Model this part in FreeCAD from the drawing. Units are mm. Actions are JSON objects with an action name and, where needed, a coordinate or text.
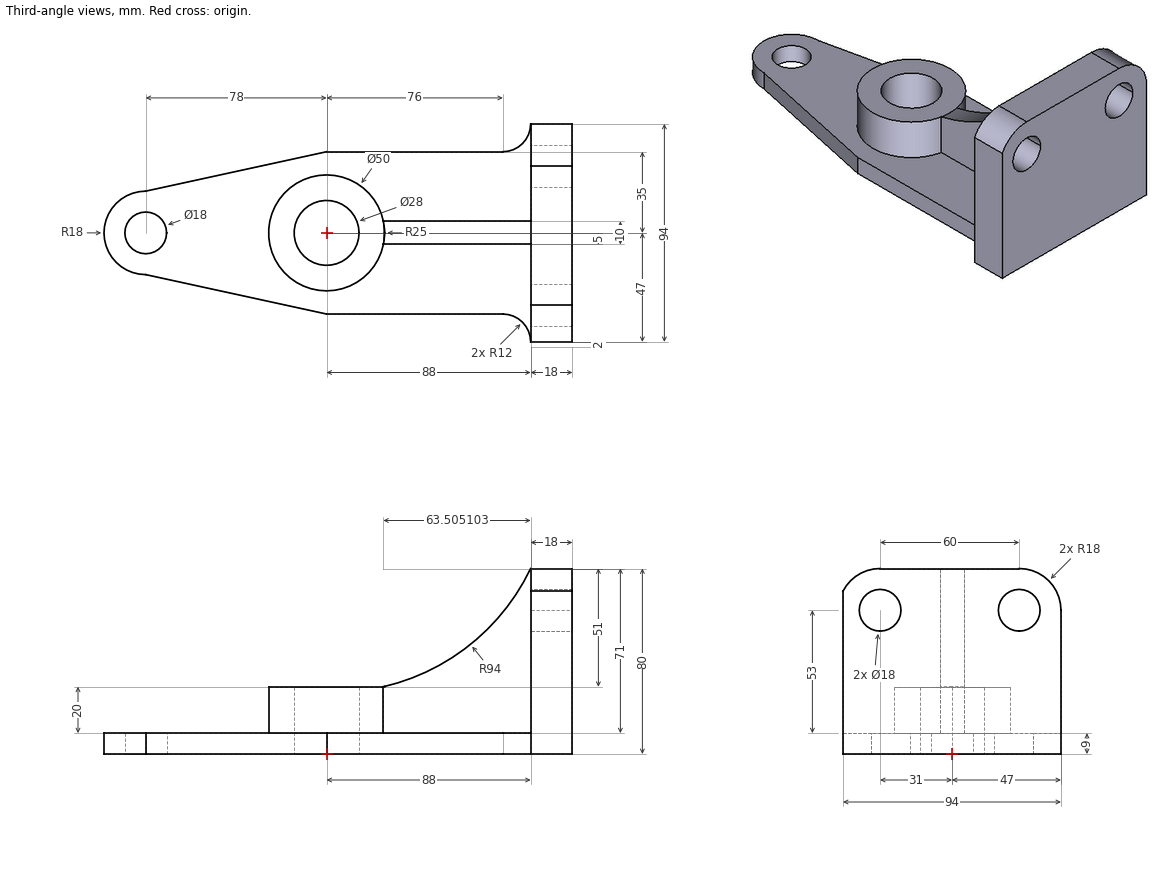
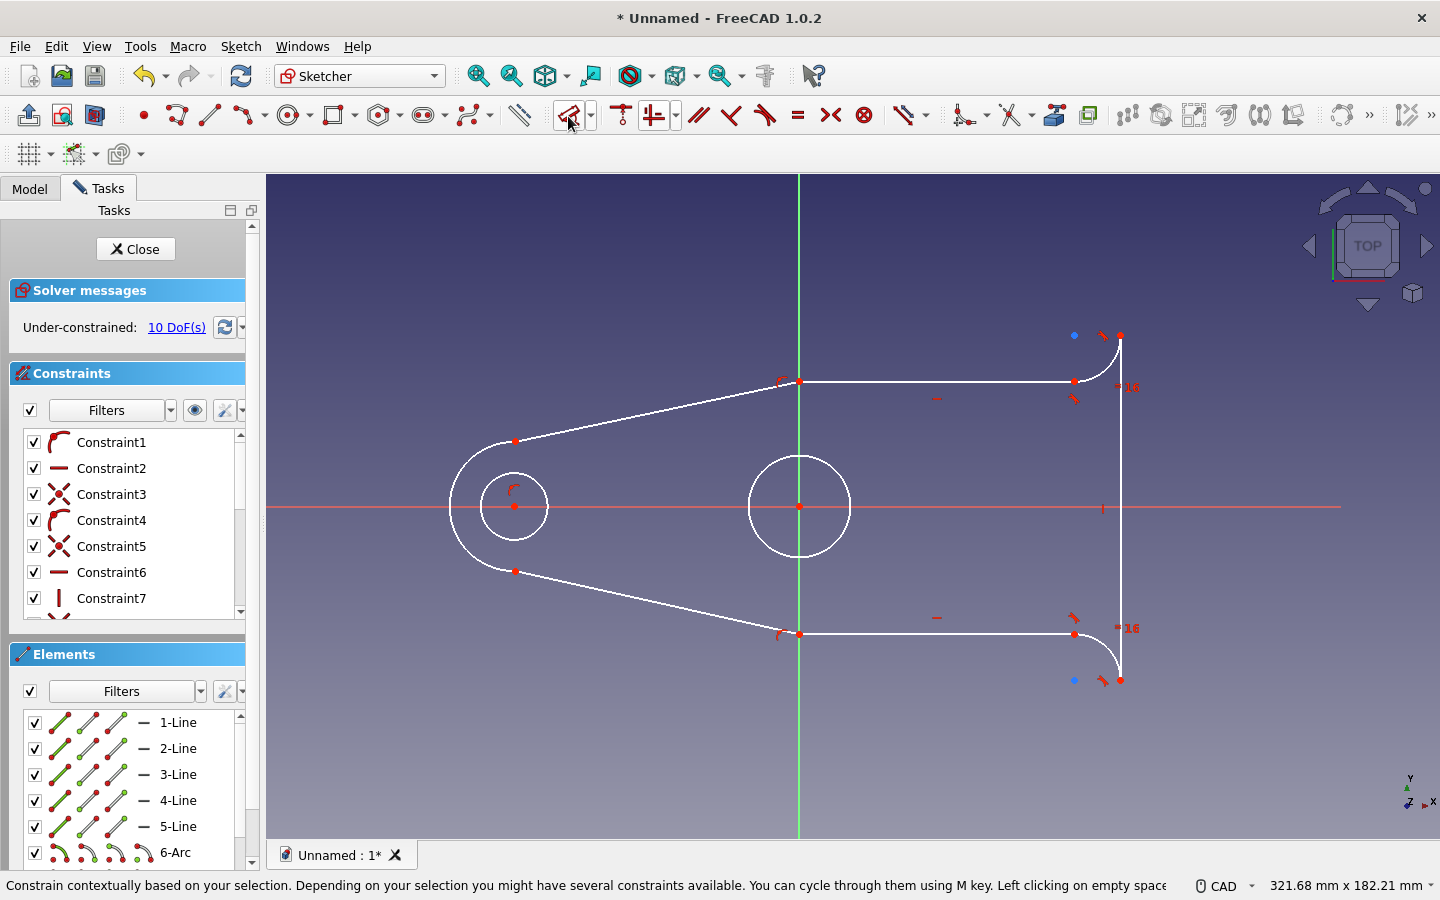
{"action": "left_click", "coordinate": [462, 468]}
{"action": "left_click", "coordinate": [436, 449]}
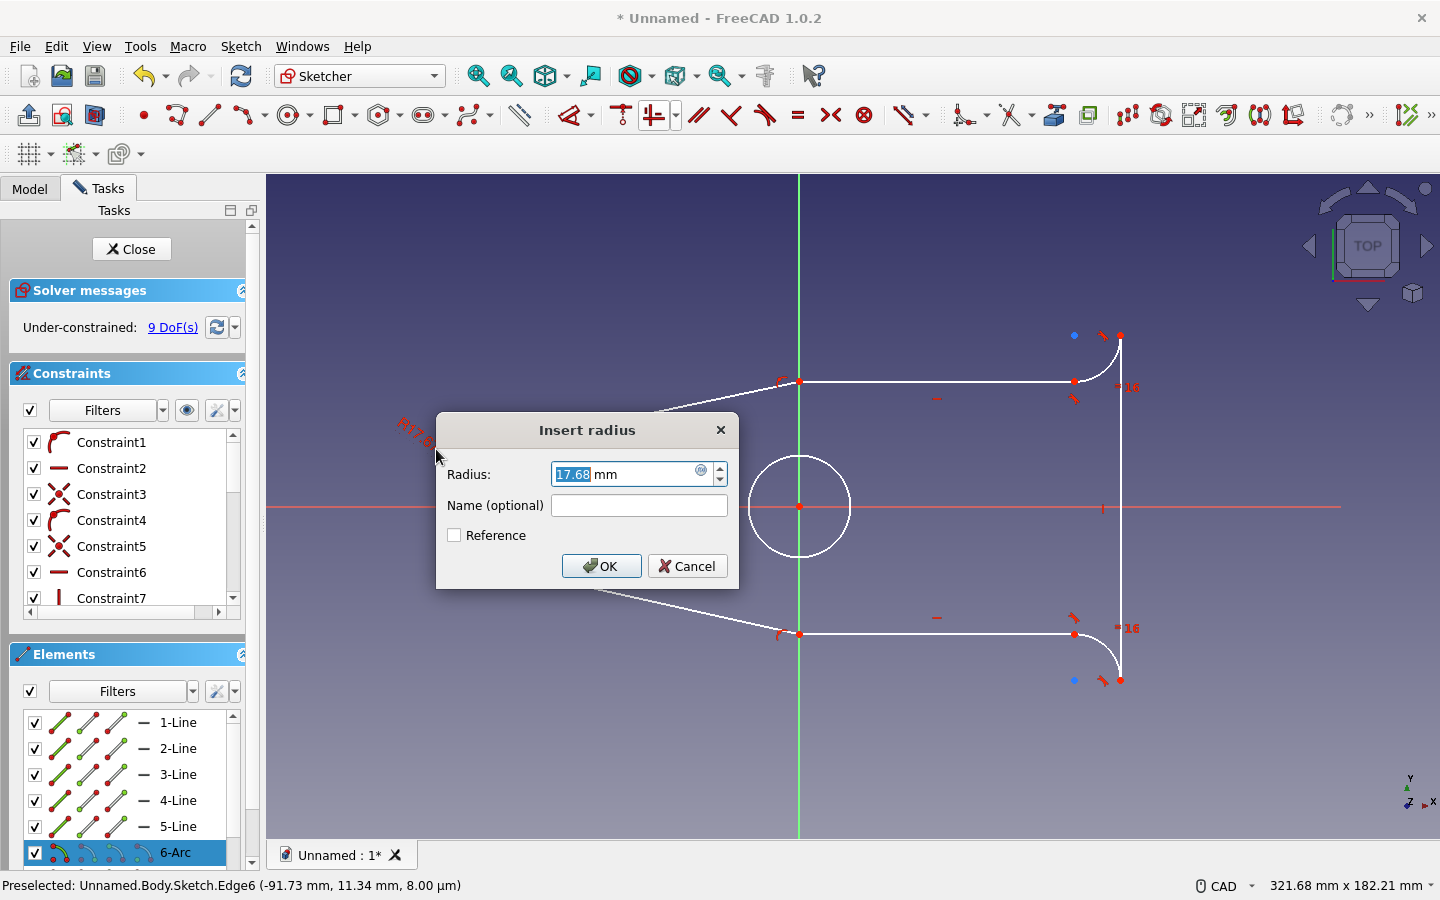
{"action": "type", "text": "18"}
{"action": "key", "text": "Return"}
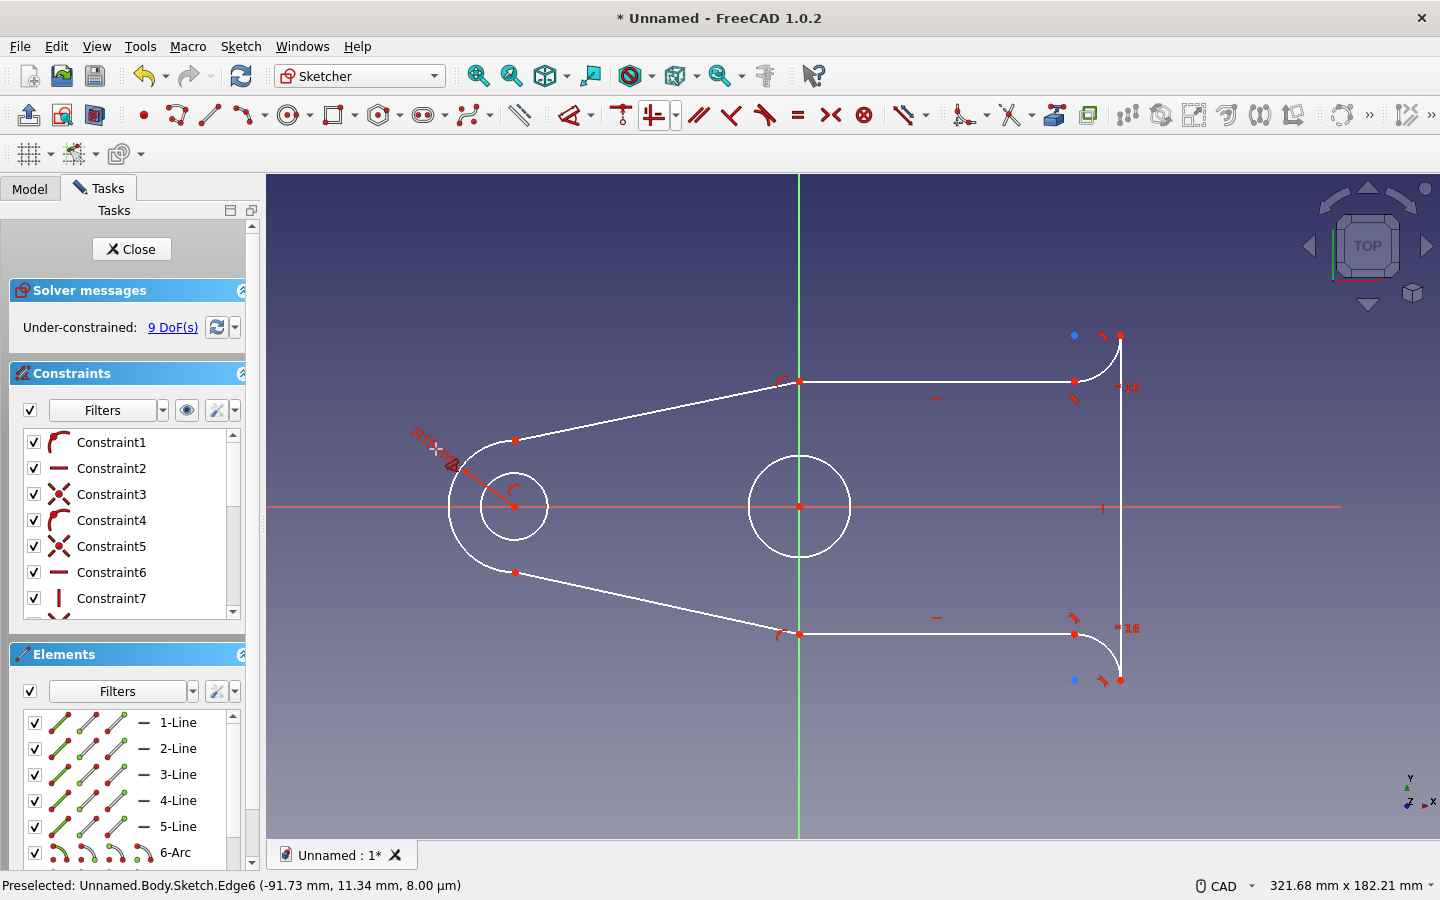
{"action": "left_click", "coordinate": [1096, 639]}
{"action": "left_click", "coordinate": [1140, 636]}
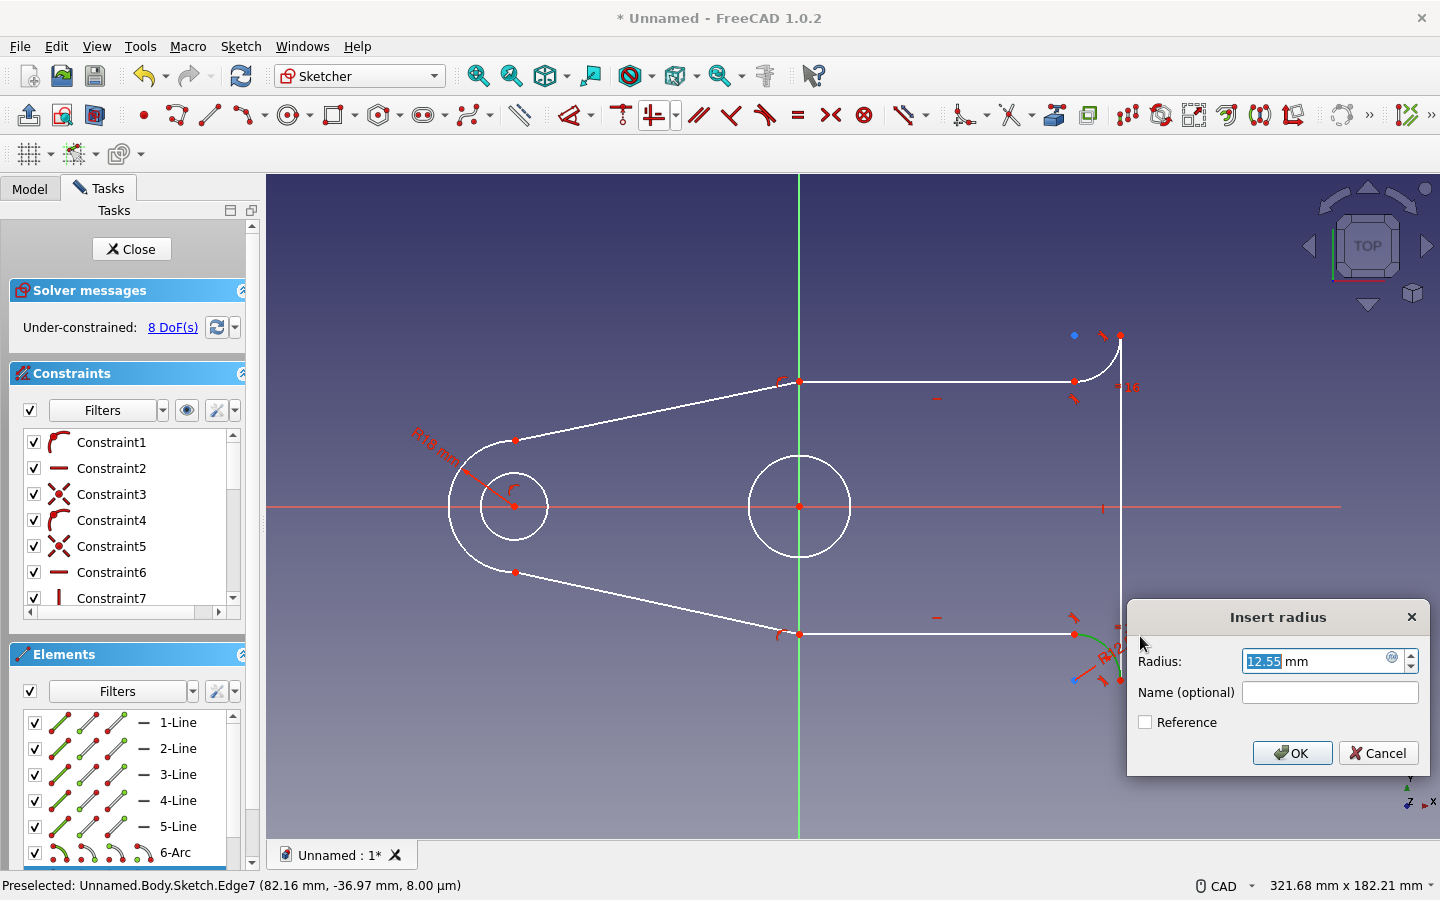
{"action": "type", "text": "12"}
{"action": "key", "text": "Return"}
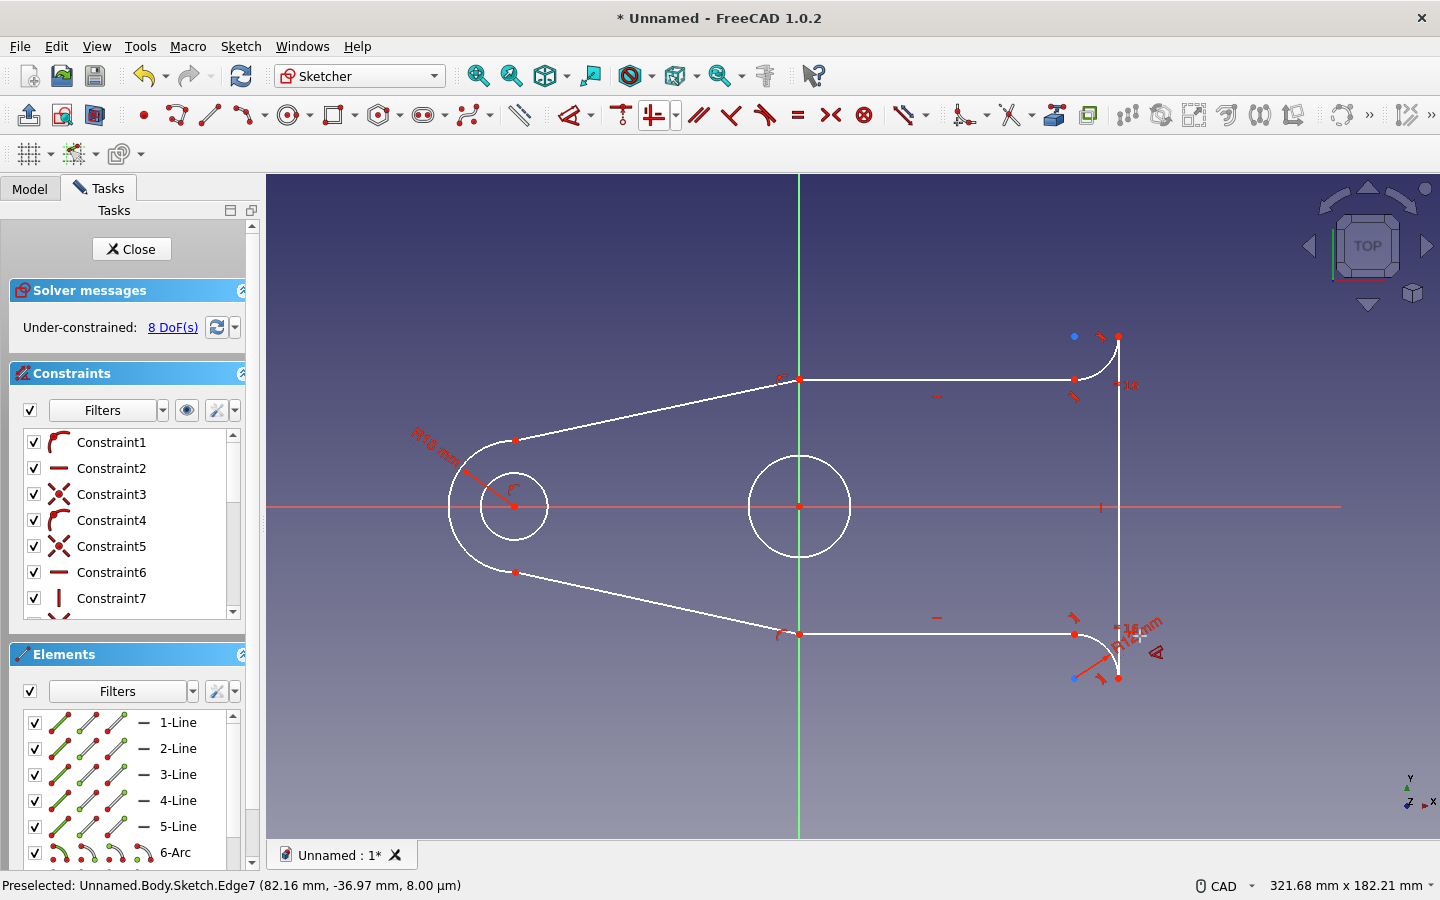
{"action": "left_click", "coordinate": [538, 483]}
{"action": "left_click", "coordinate": [561, 461]}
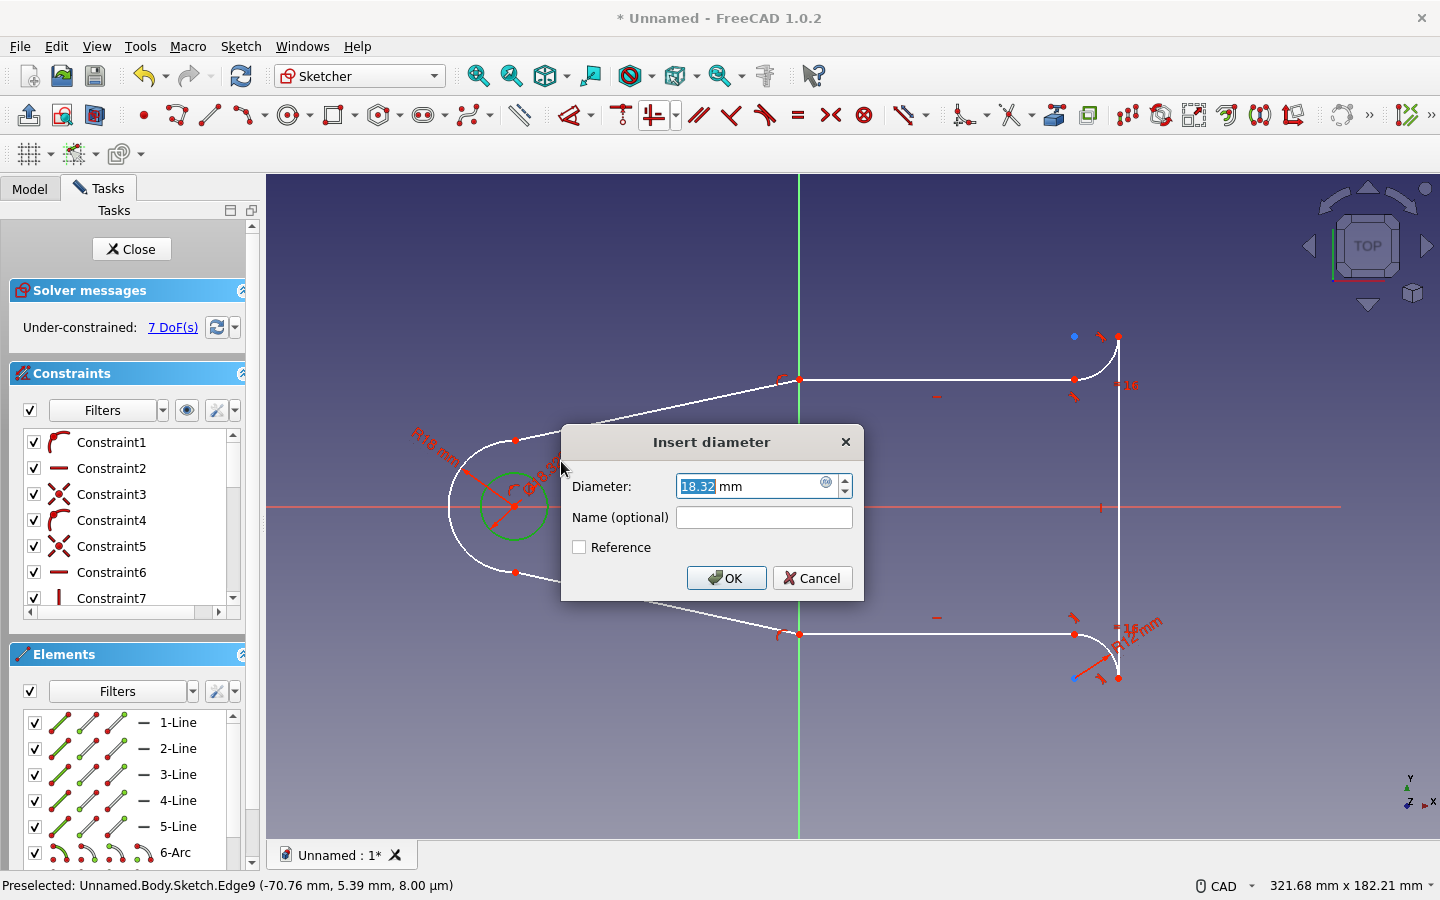
{"action": "type", "text": "18"}
{"action": "key", "text": "Return"}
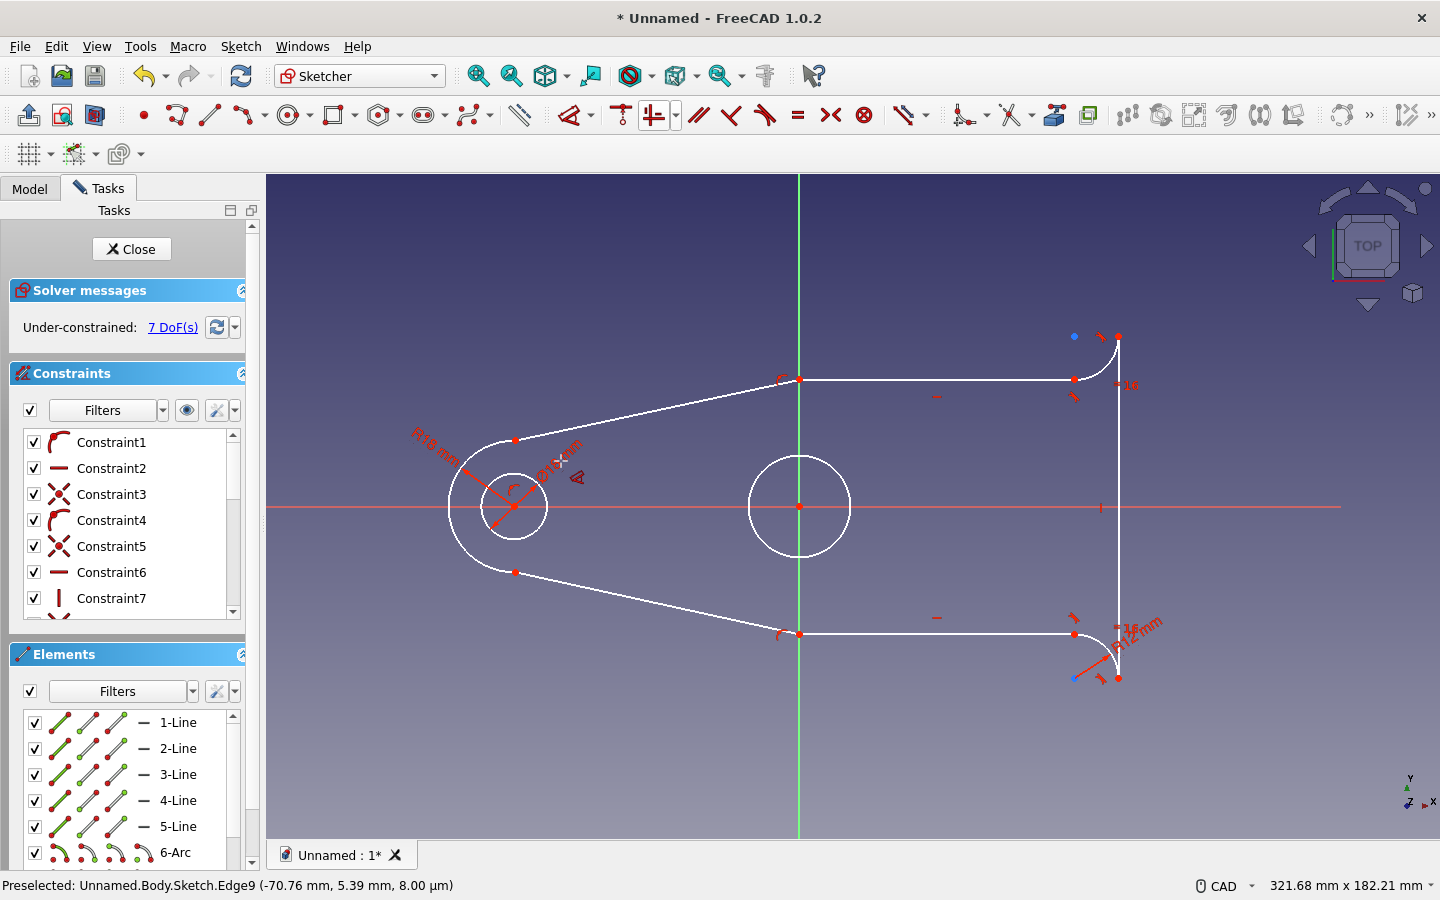
{"action": "left_click", "coordinate": [835, 470]}
{"action": "left_click", "coordinate": [857, 447]}